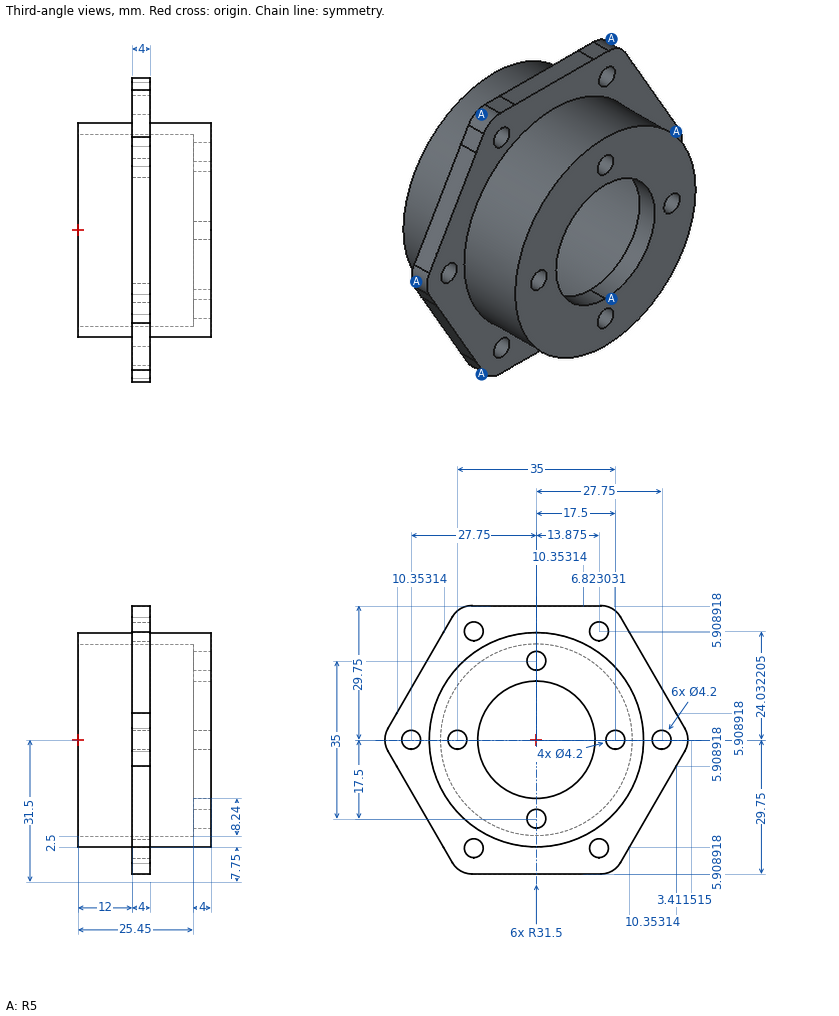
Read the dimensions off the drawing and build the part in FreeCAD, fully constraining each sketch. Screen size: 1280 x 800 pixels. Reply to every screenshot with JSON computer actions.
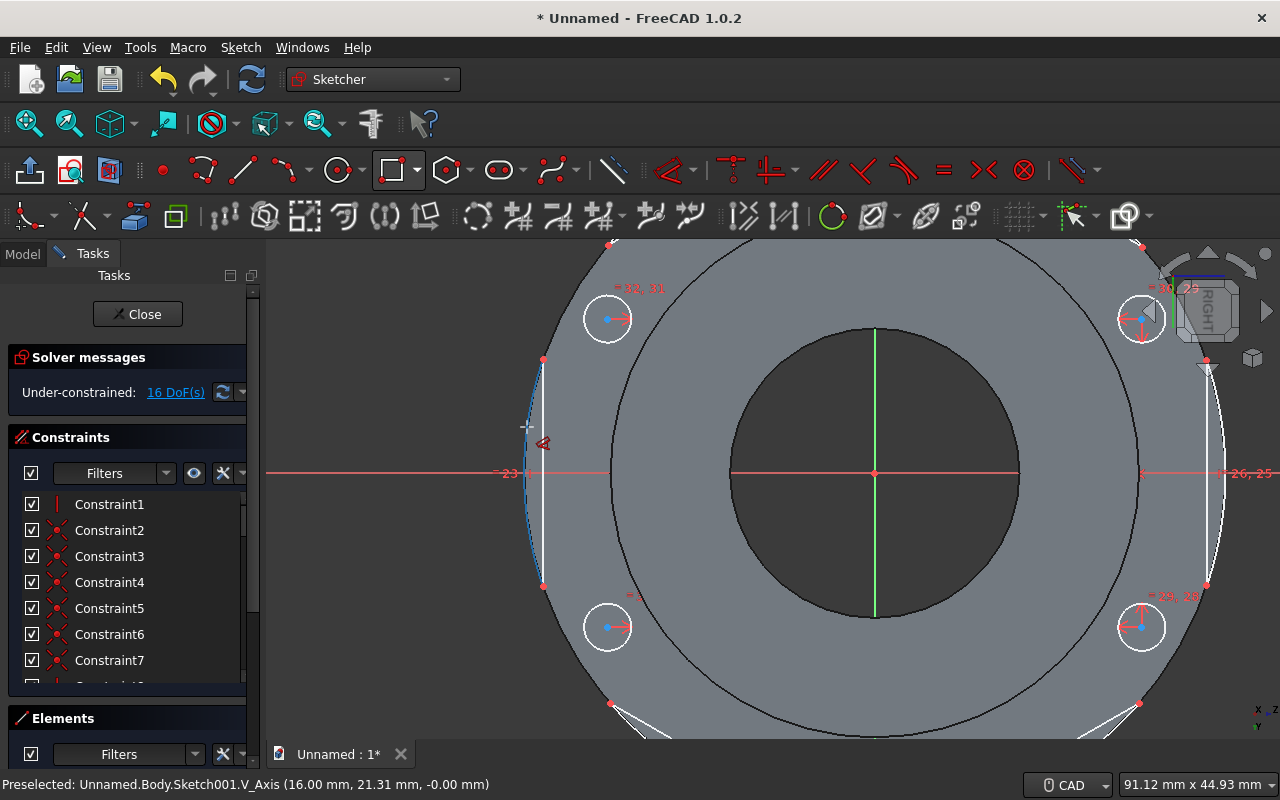
{"action": "left_click", "coordinate": [527, 427]}
{"action": "left_click", "coordinate": [495, 423]}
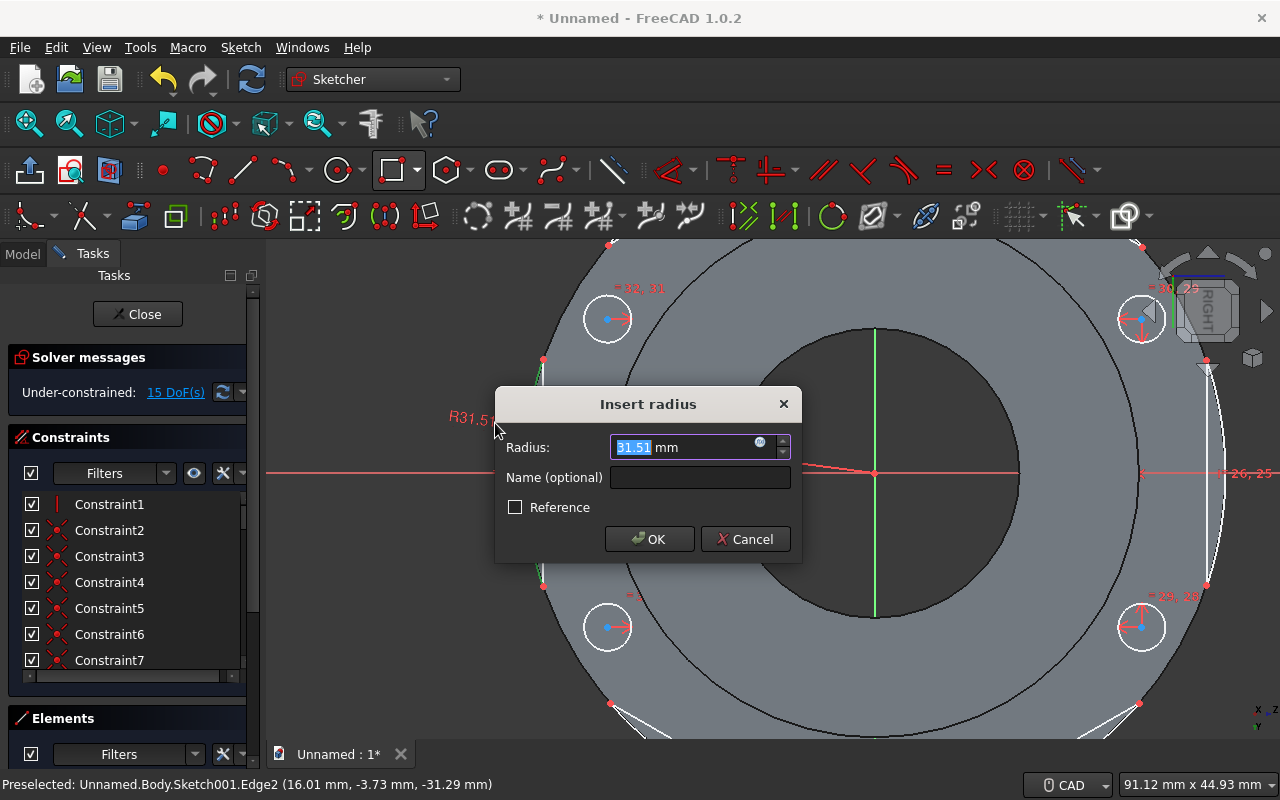
{"action": "type", "text": "31.5"}
{"action": "key", "text": "Return"}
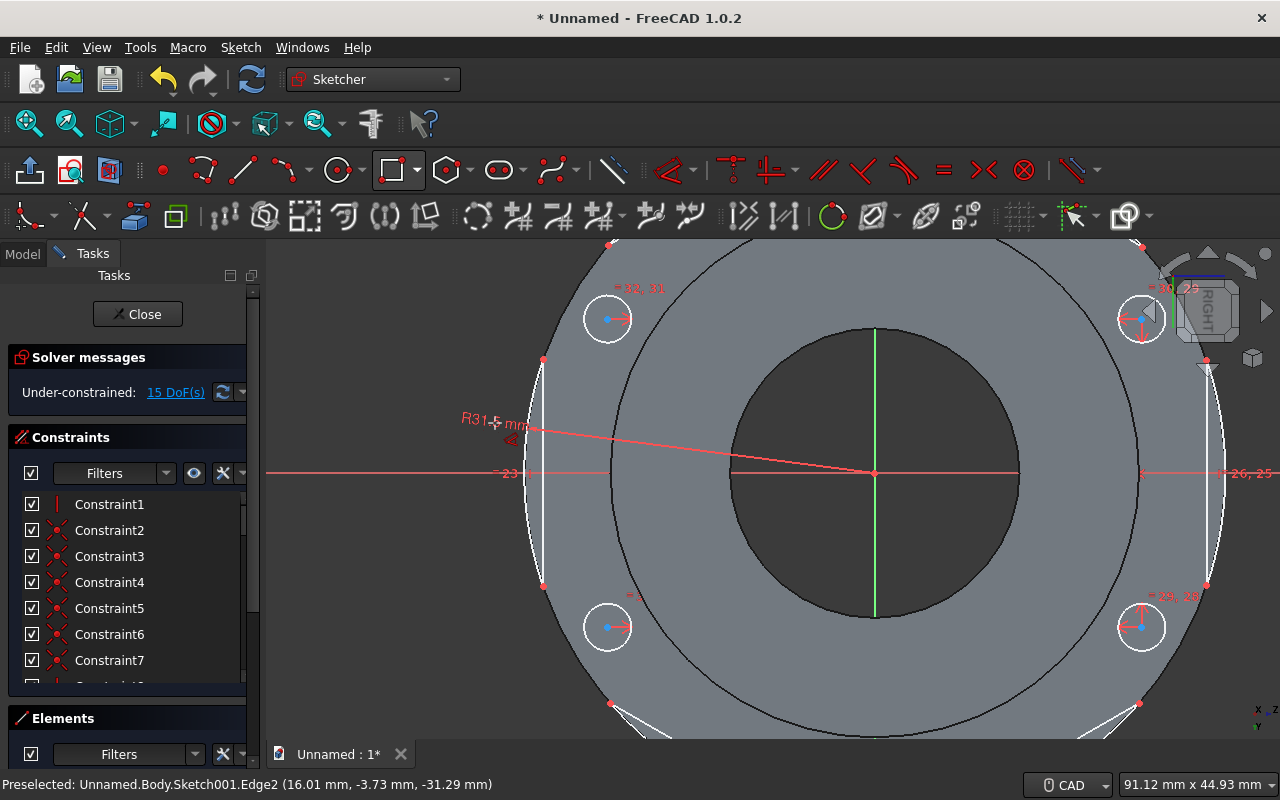
{"action": "scroll", "coordinate": [566, 502], "scroll_direction": "down", "scroll_amount": 4}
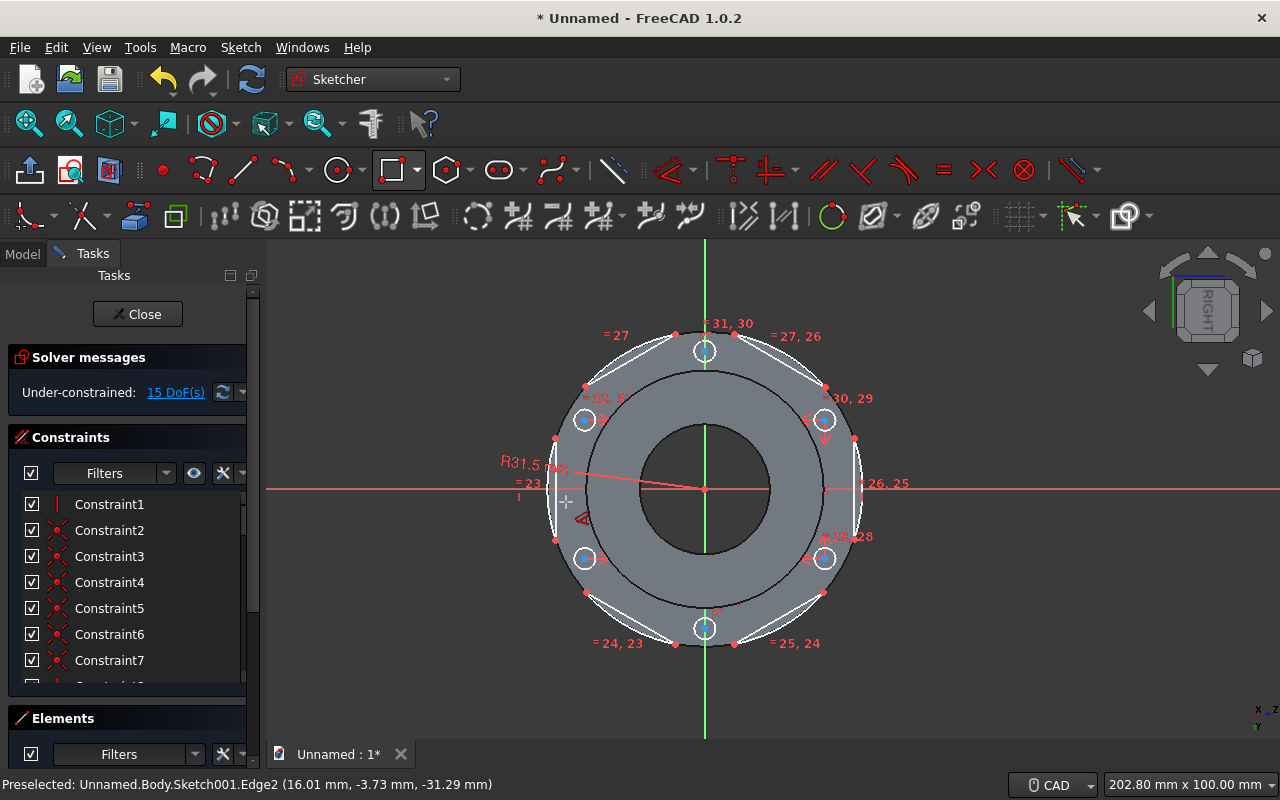
{"action": "scroll", "coordinate": [712, 621], "scroll_direction": "up", "scroll_amount": 4}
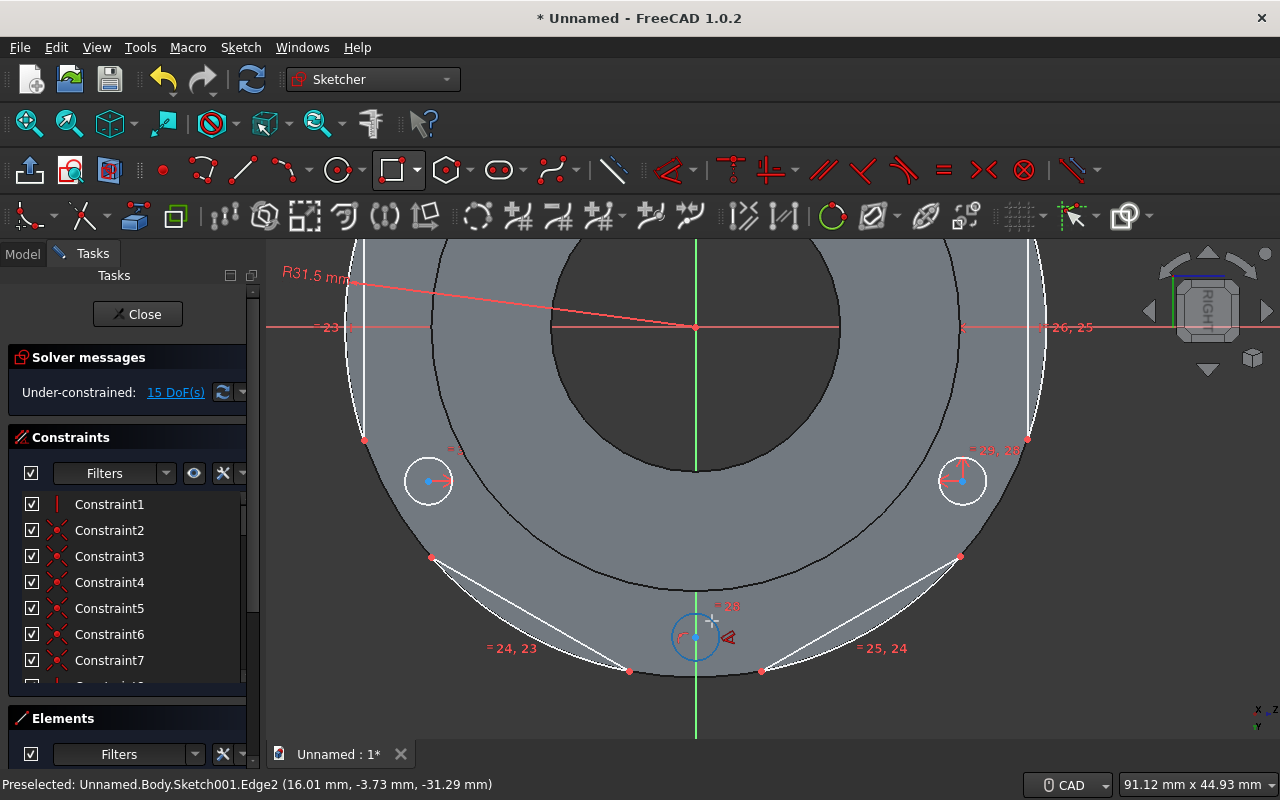
{"action": "left_click", "coordinate": [712, 620]}
{"action": "left_click", "coordinate": [734, 597]}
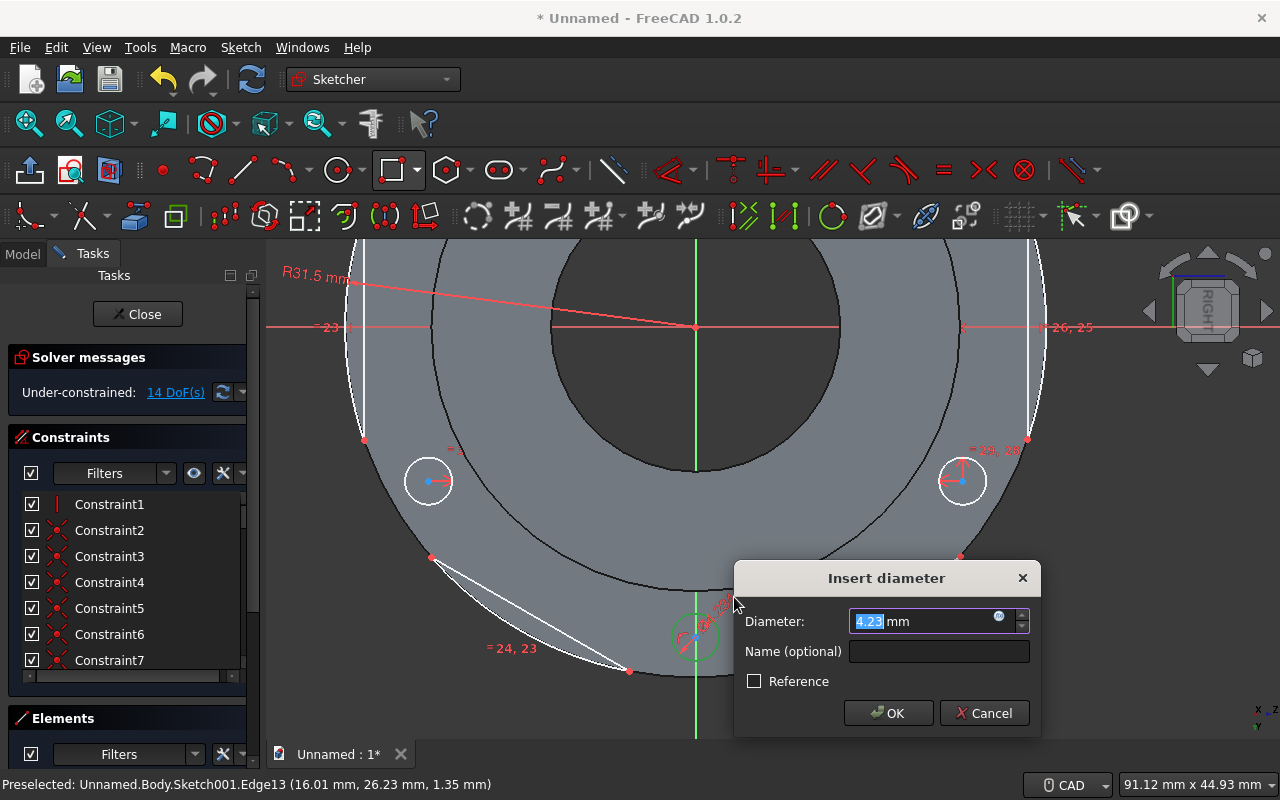
{"action": "type", "text": "4.2"}
{"action": "key", "text": "Return"}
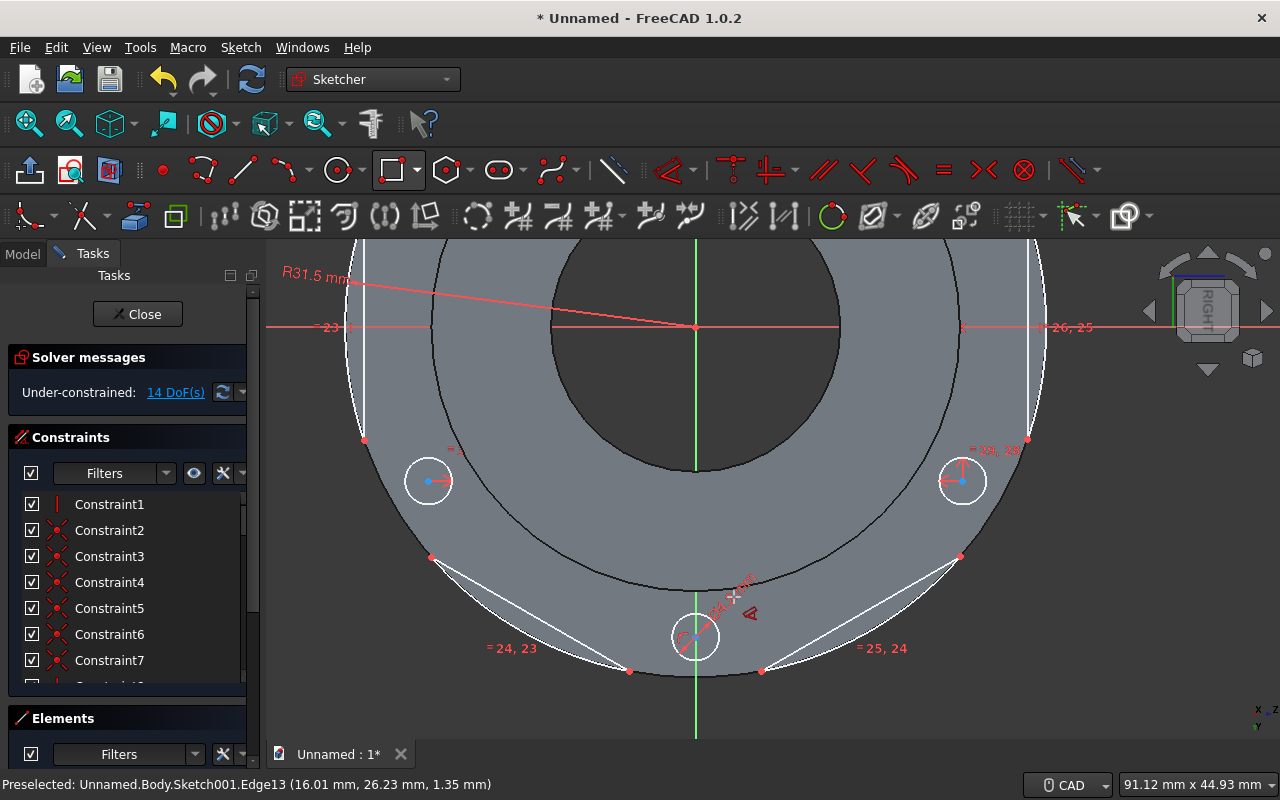
{"action": "left_click", "coordinate": [696, 637]}
{"action": "left_click", "coordinate": [730, 482]}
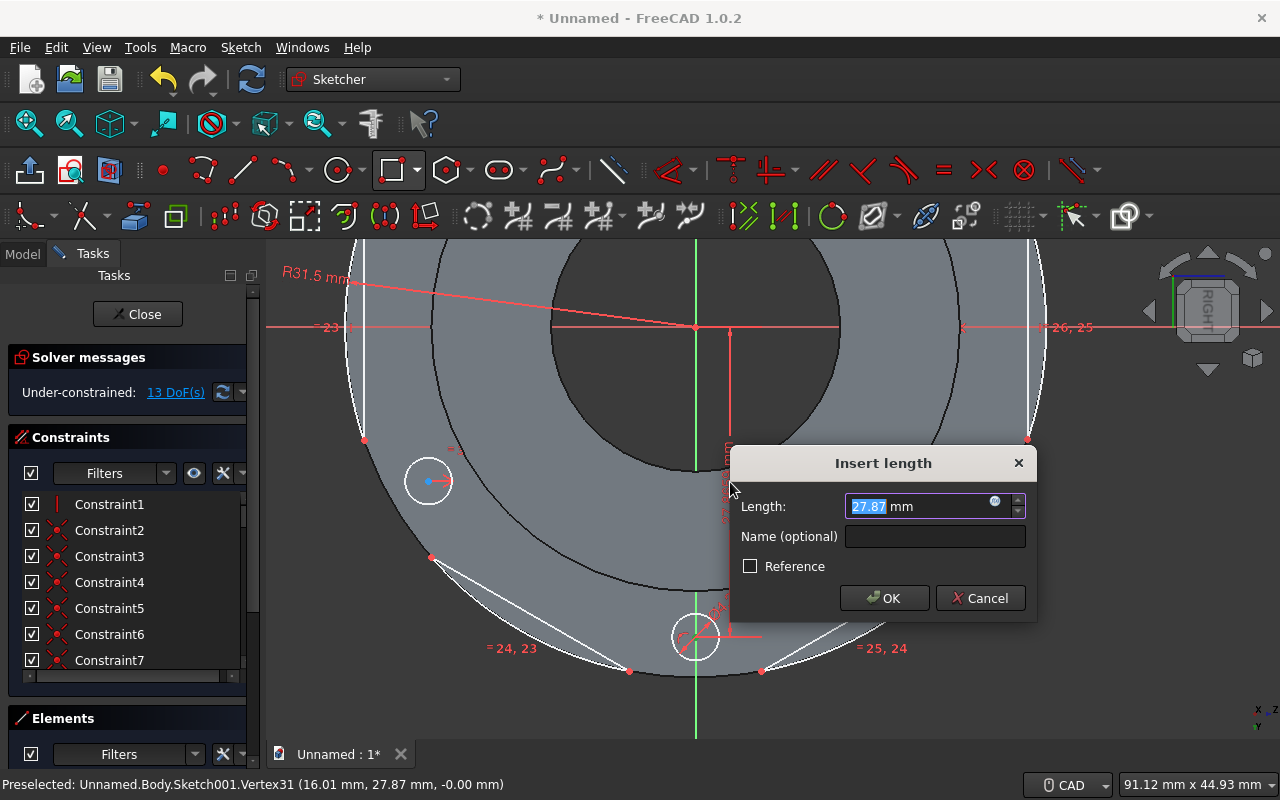
{"action": "type", "text": "27.75"}
{"action": "key", "text": "Return"}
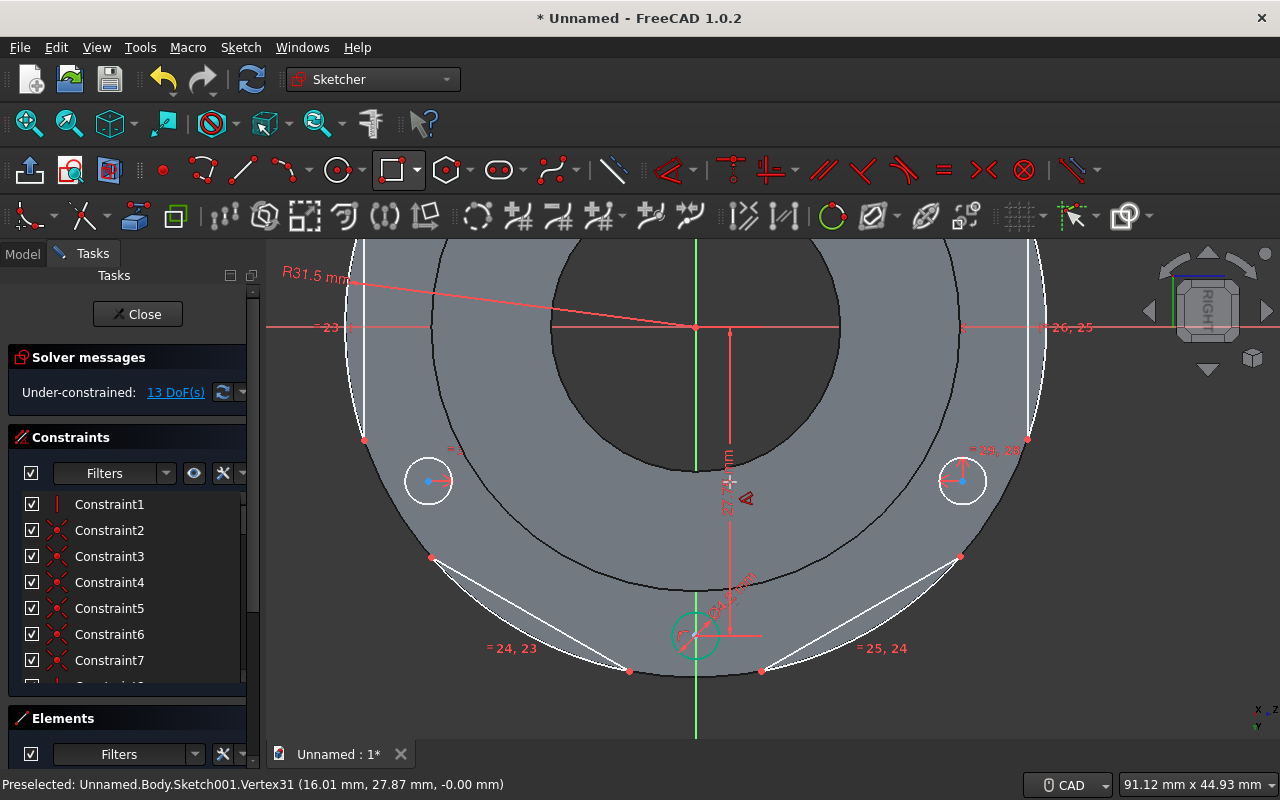
{"action": "scroll", "coordinate": [712, 621], "scroll_direction": "down", "scroll_amount": 4}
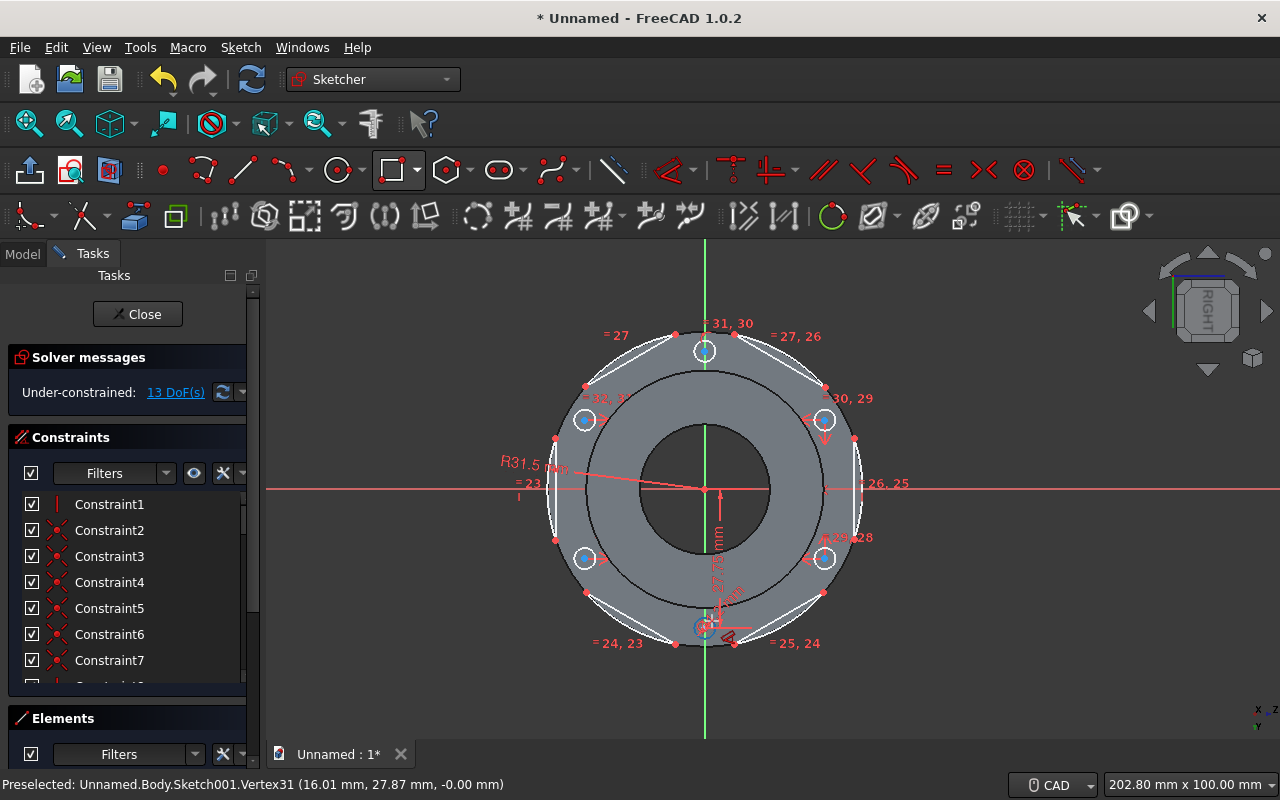
{"action": "left_click", "coordinate": [705, 351]}
{"action": "left_click", "coordinate": [739, 420]}